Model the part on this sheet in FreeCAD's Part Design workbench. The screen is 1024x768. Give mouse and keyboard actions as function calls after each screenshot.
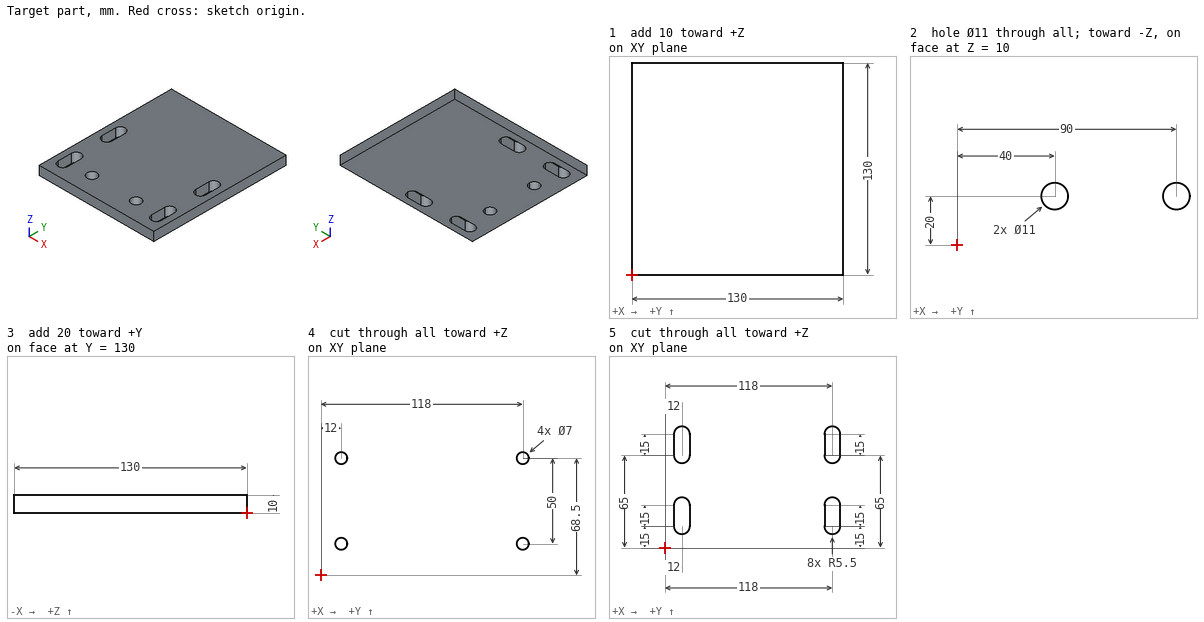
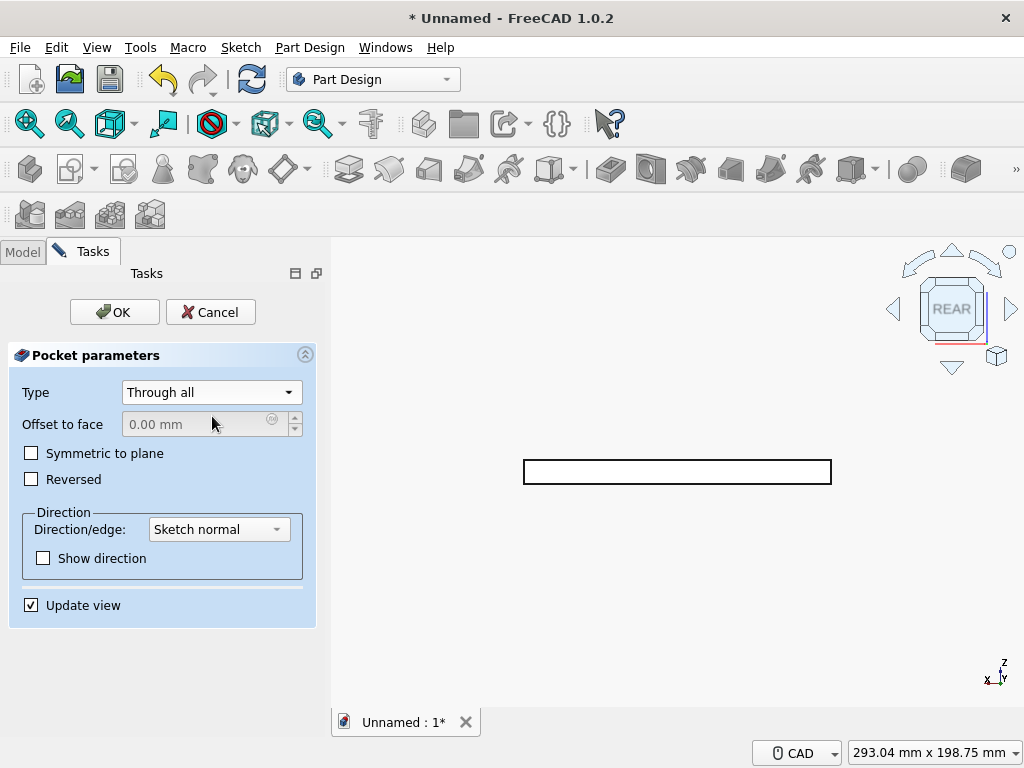
click(30, 479)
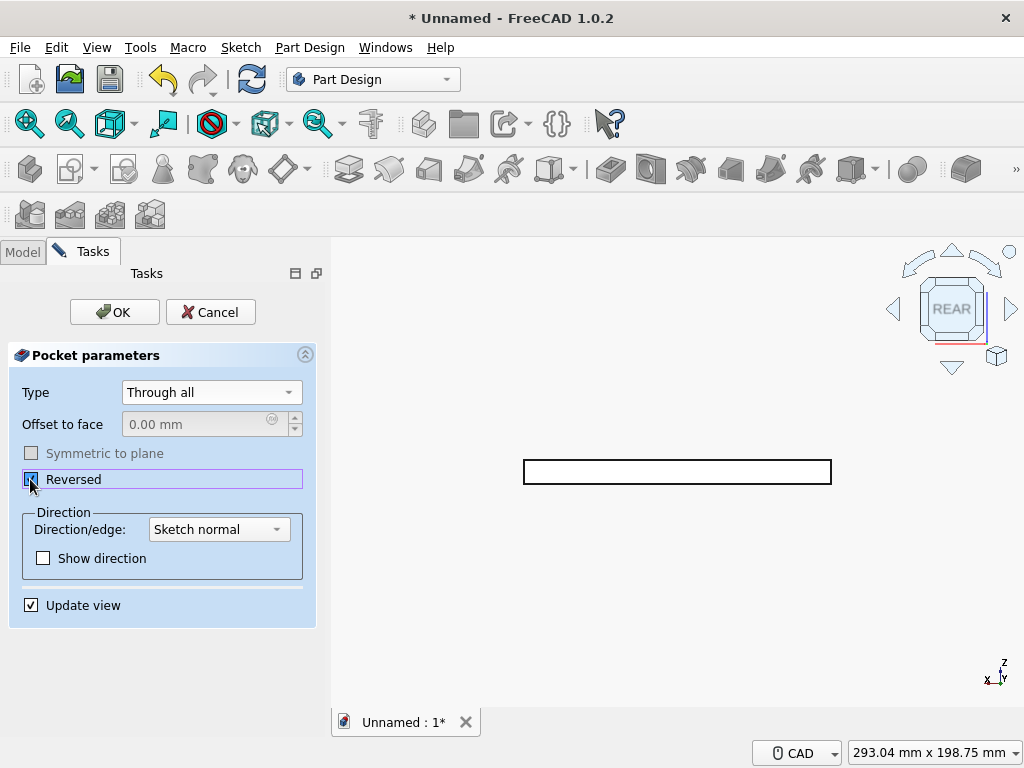
click(115, 312)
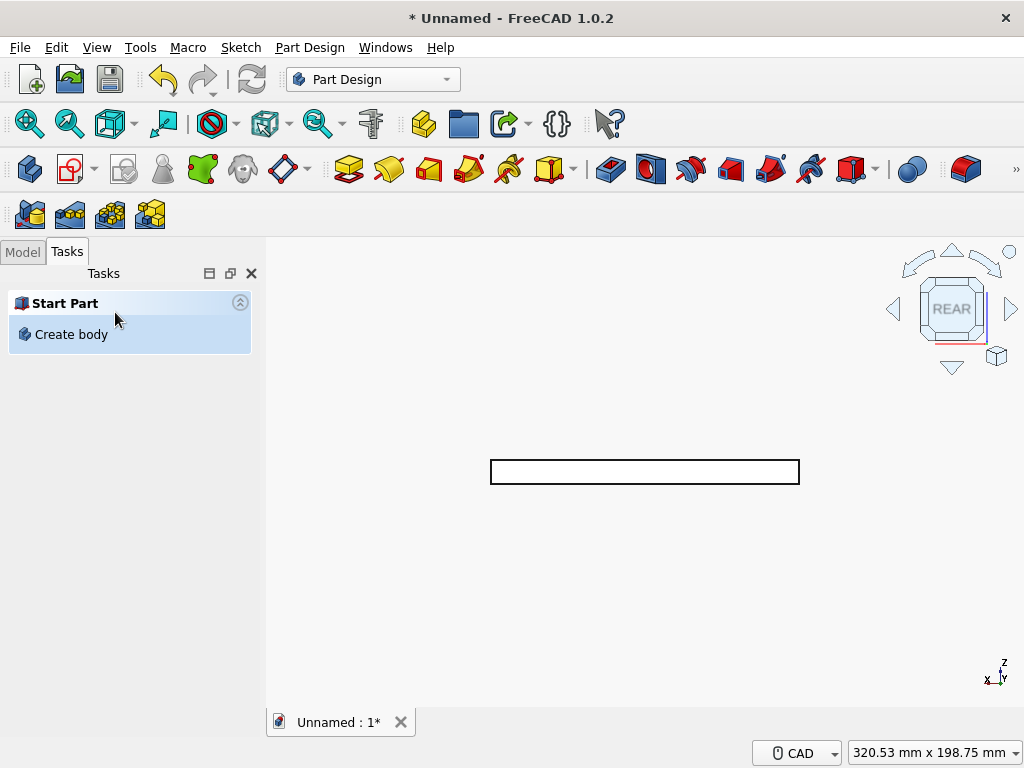
key(0)